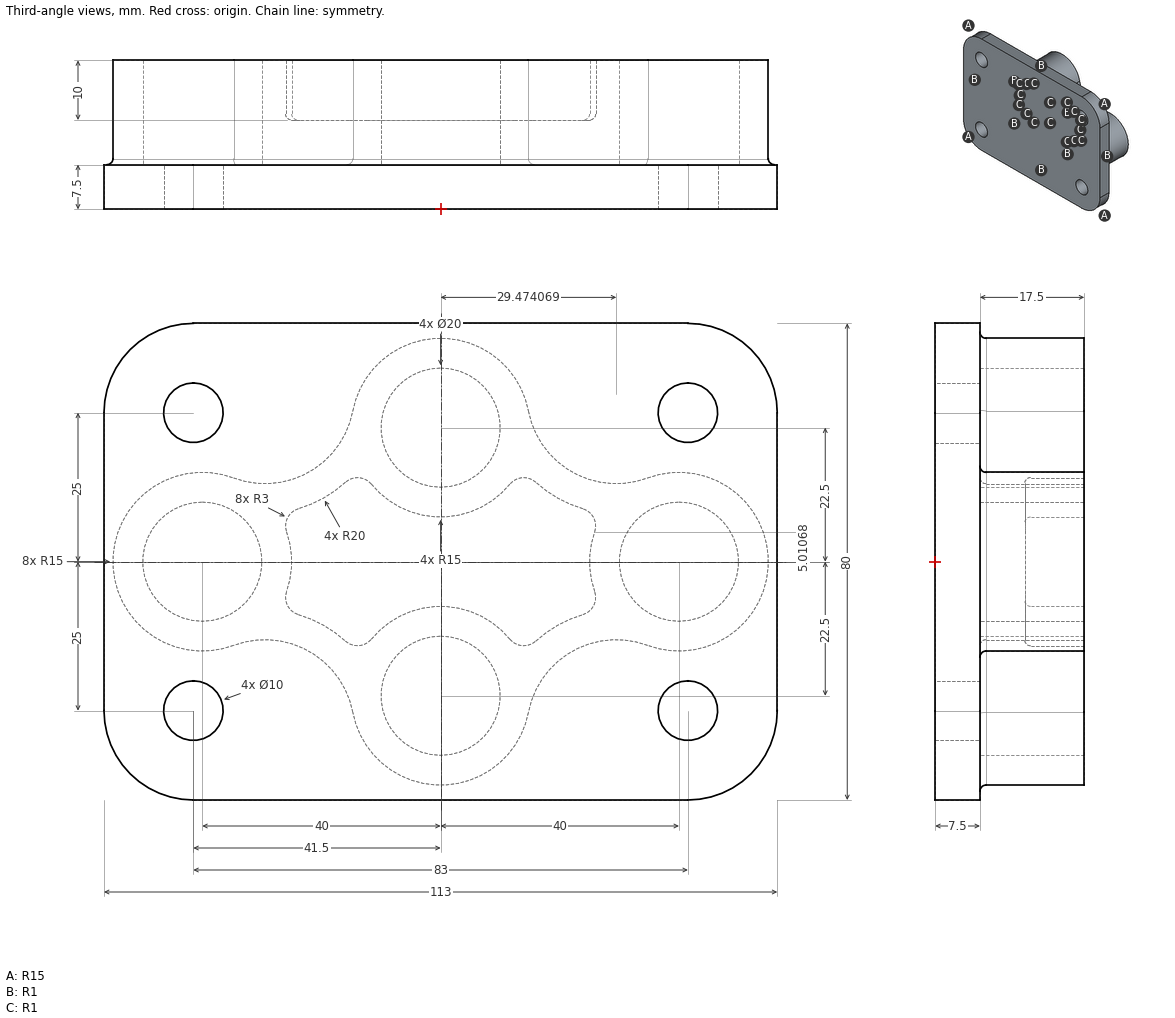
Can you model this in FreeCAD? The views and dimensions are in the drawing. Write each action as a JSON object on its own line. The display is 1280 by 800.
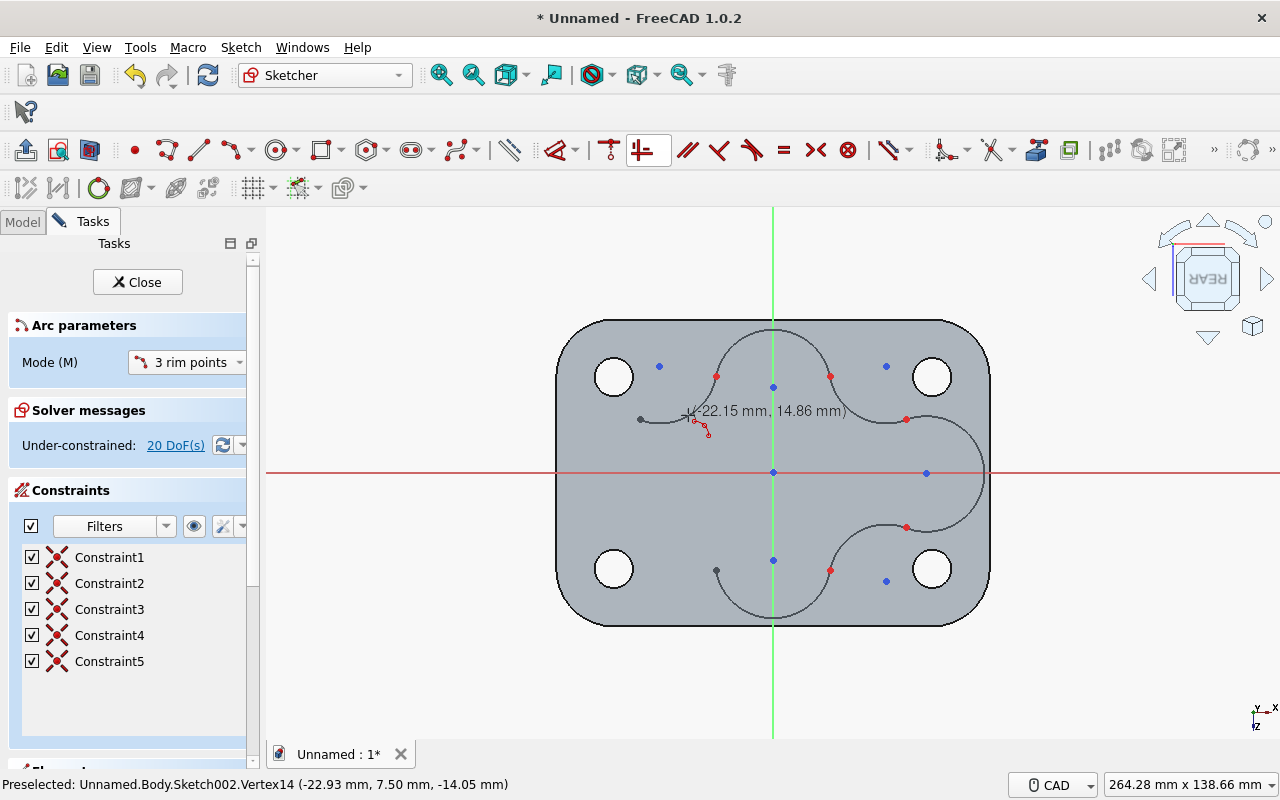
{"action": "left_click", "coordinate": [640, 420]}
{"action": "left_click", "coordinate": [640, 527]}
{"action": "left_click", "coordinate": [566, 451]}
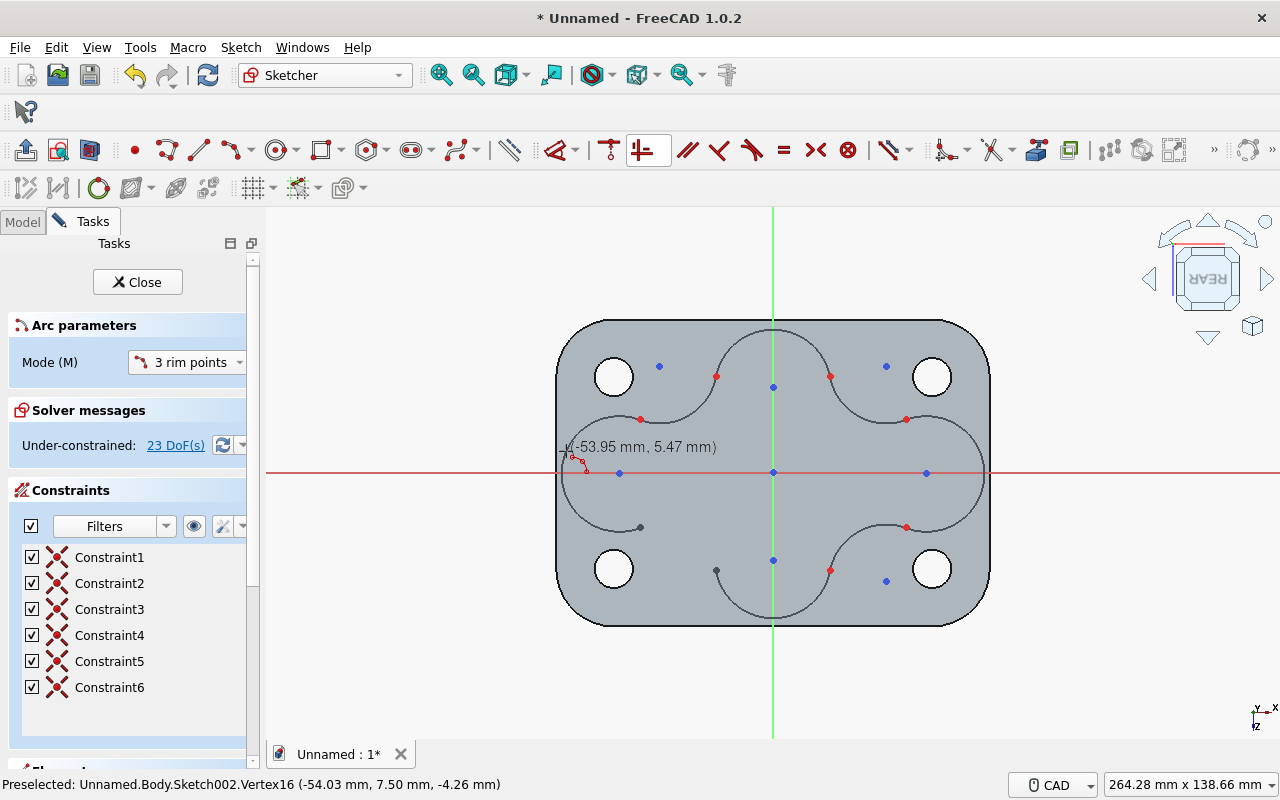
{"action": "left_click", "coordinate": [640, 528]}
{"action": "left_click", "coordinate": [716, 571]}
{"action": "left_click", "coordinate": [688, 531]}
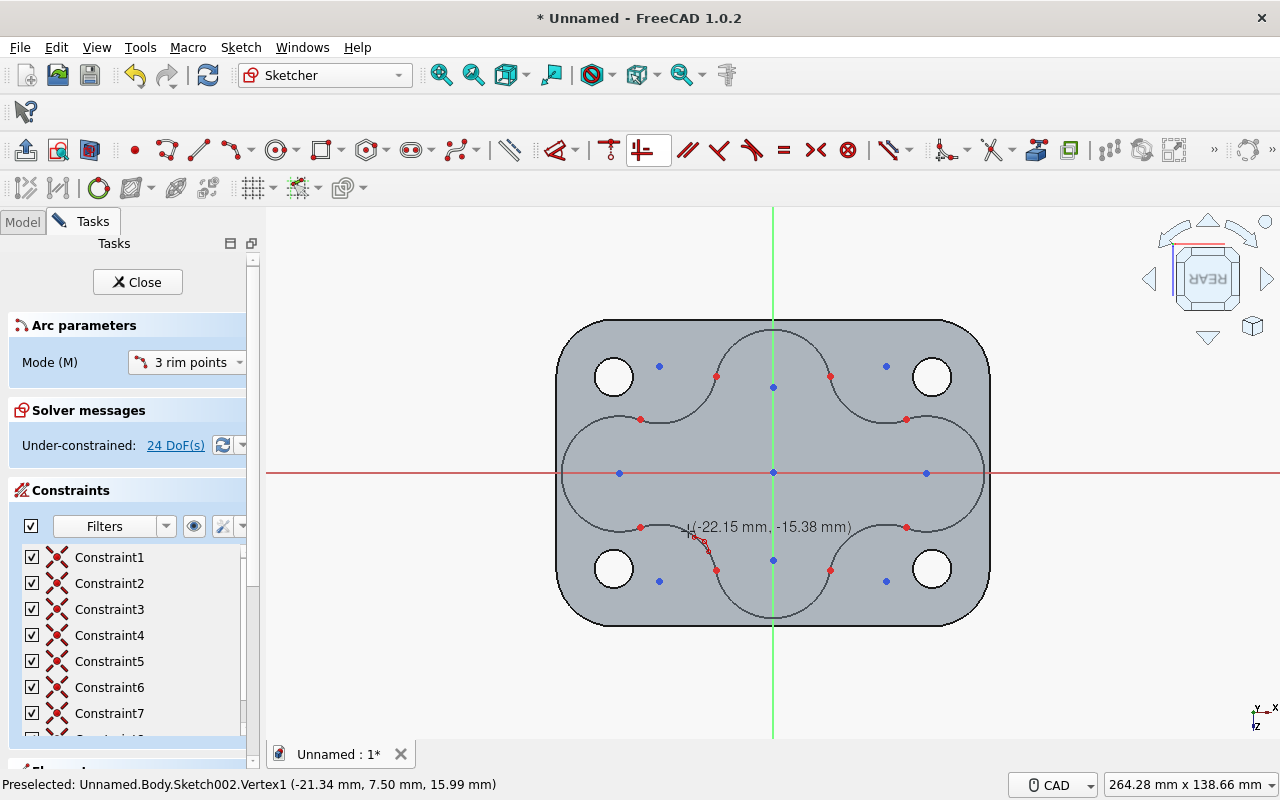
{"action": "key", "text": "g c"}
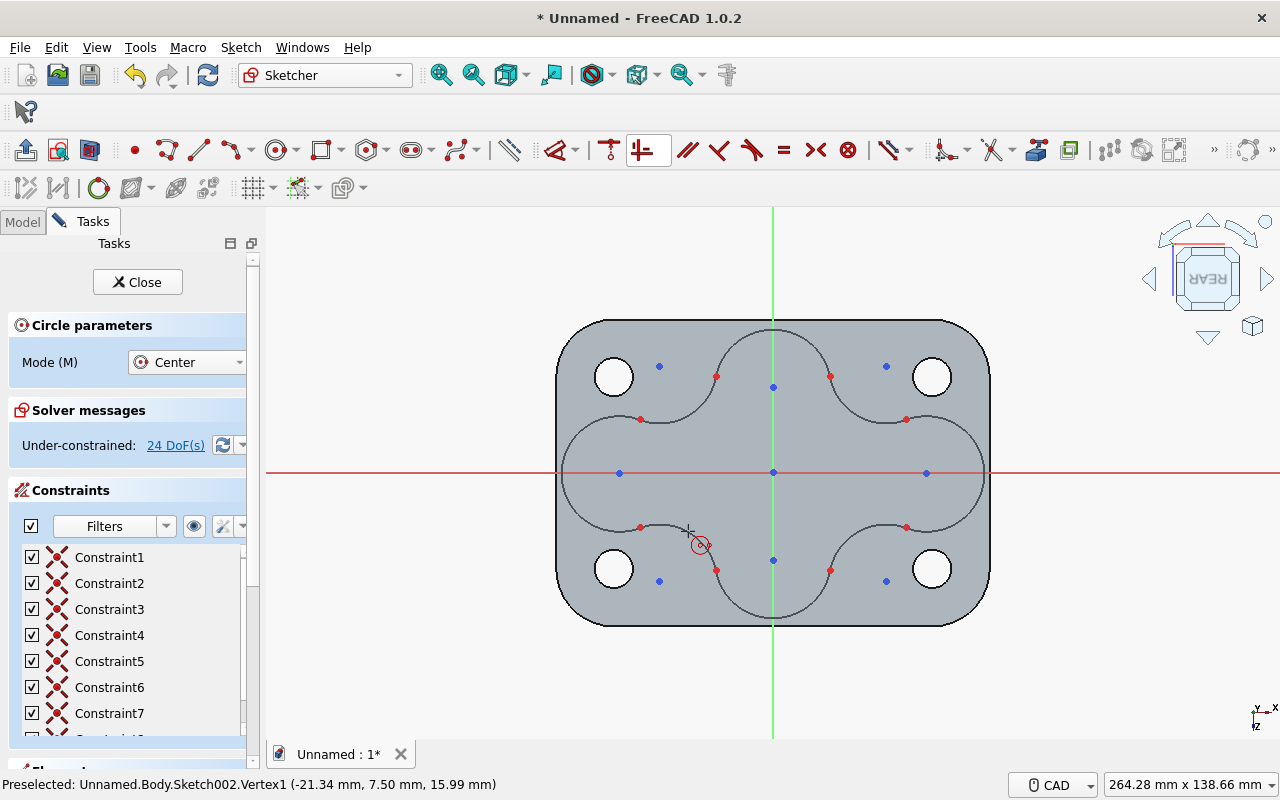
{"action": "left_click", "coordinate": [773, 559]}
{"action": "mouse_move", "coordinate": [800, 532]}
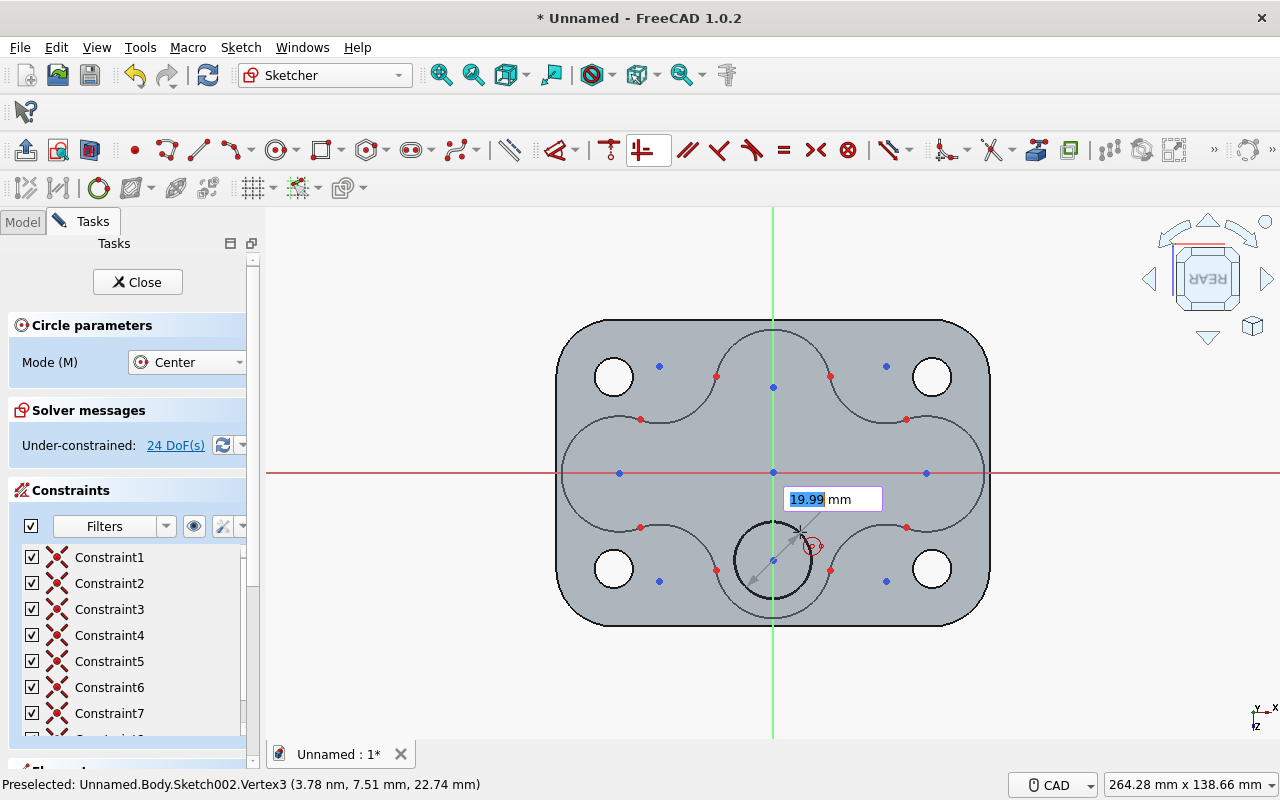
{"action": "type", "text": "20"}
{"action": "key", "text": "Return"}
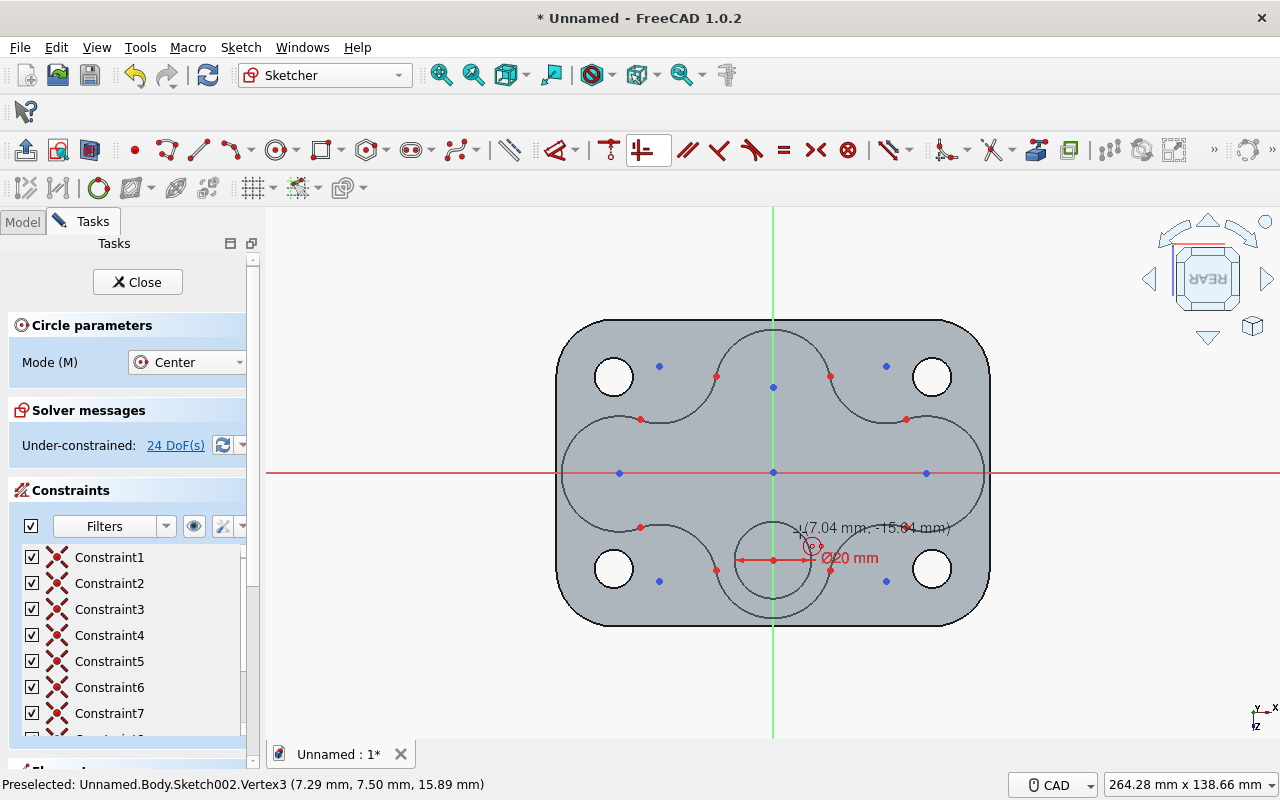
{"action": "left_click", "coordinate": [620, 473]}
{"action": "mouse_move", "coordinate": [647, 446]}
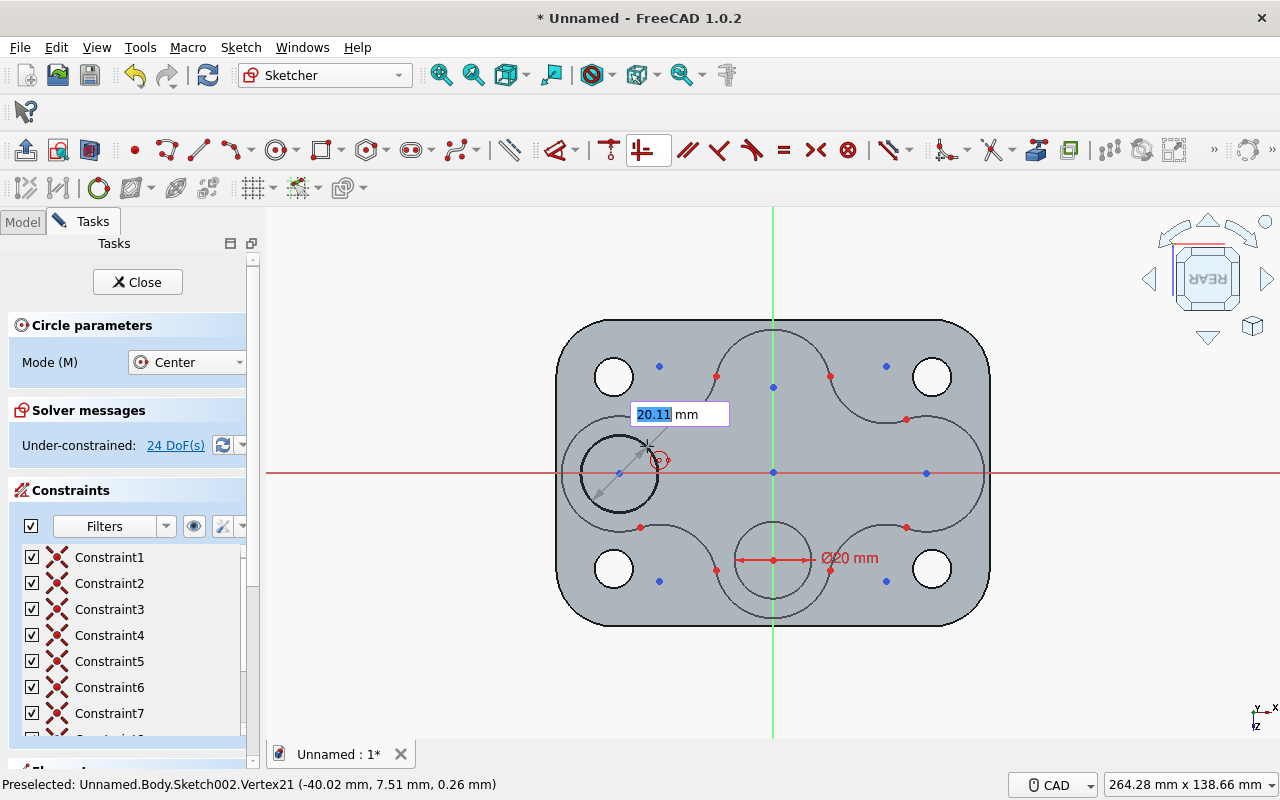
{"action": "type", "text": "20"}
{"action": "key", "text": "Return"}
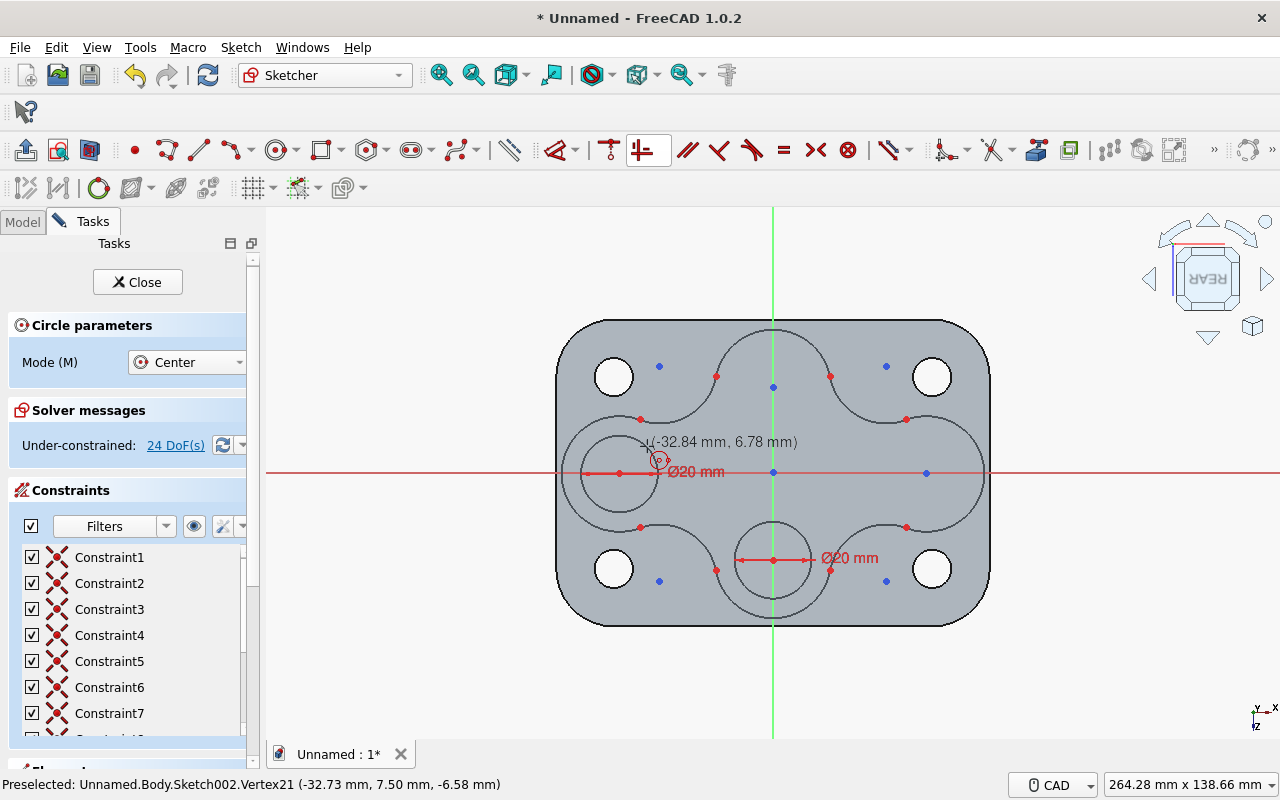
{"action": "left_click", "coordinate": [926, 473]}
{"action": "mouse_move", "coordinate": [954, 446]}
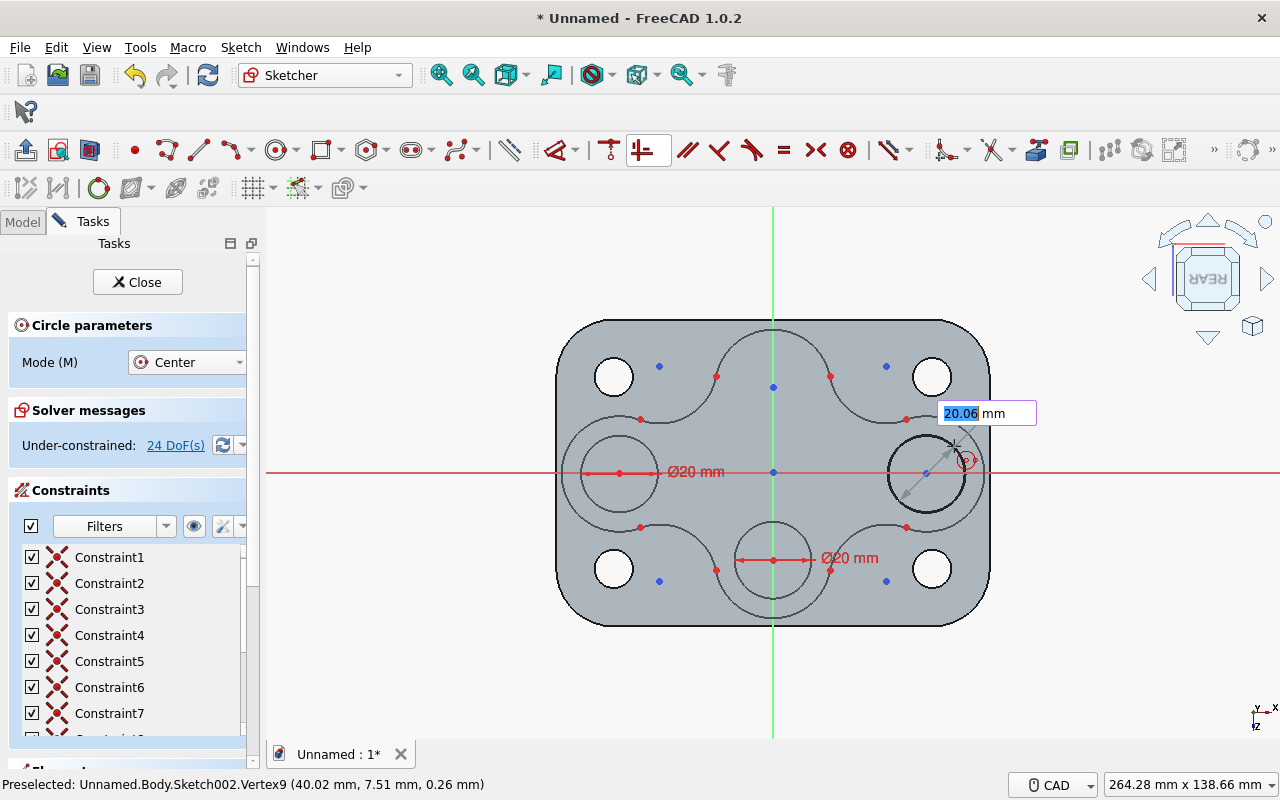
{"action": "type", "text": "20"}
{"action": "key", "text": "Return"}